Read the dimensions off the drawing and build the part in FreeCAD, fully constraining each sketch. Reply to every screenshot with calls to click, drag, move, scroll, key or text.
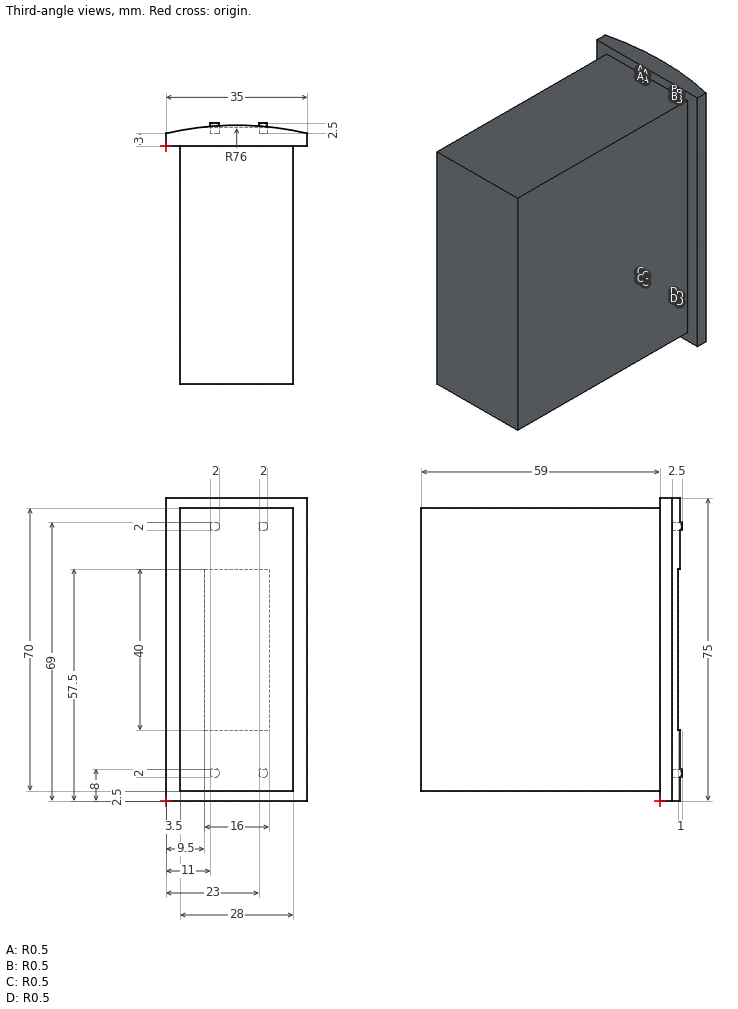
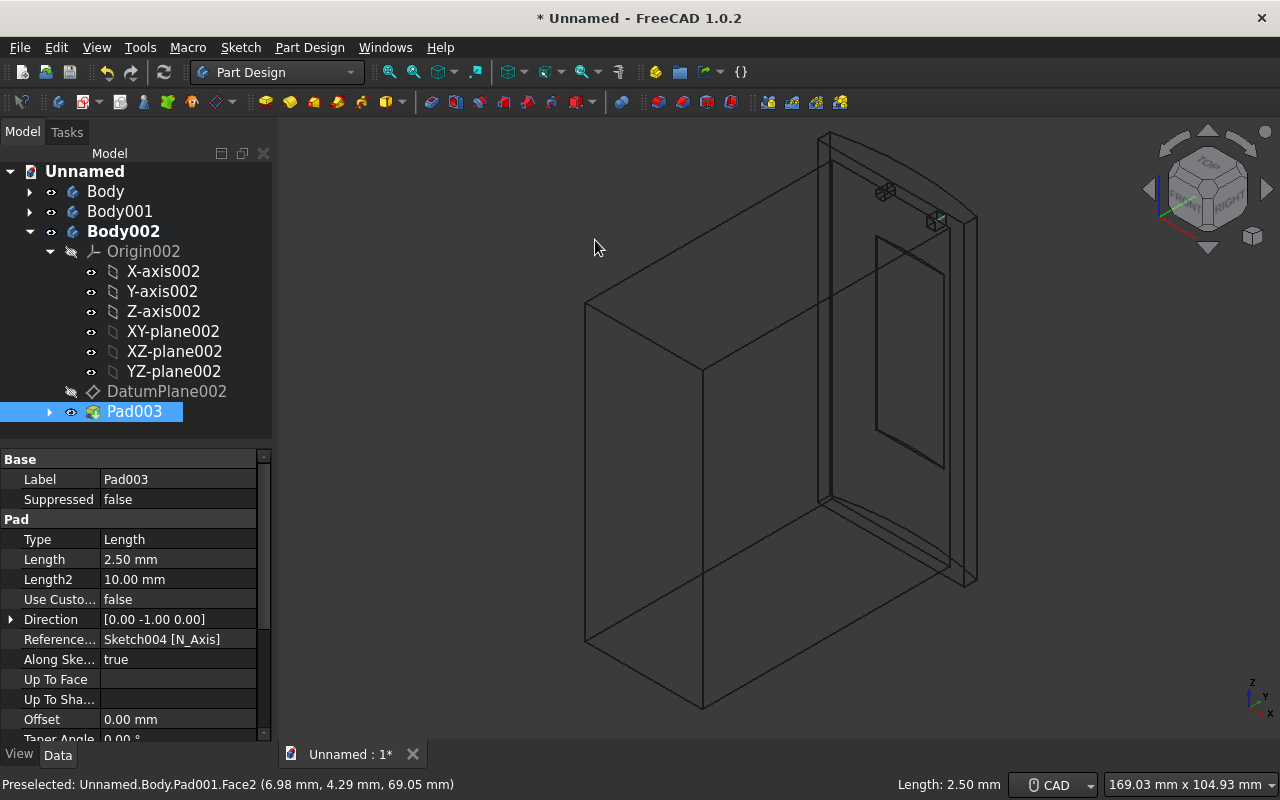
key(v)
key(f)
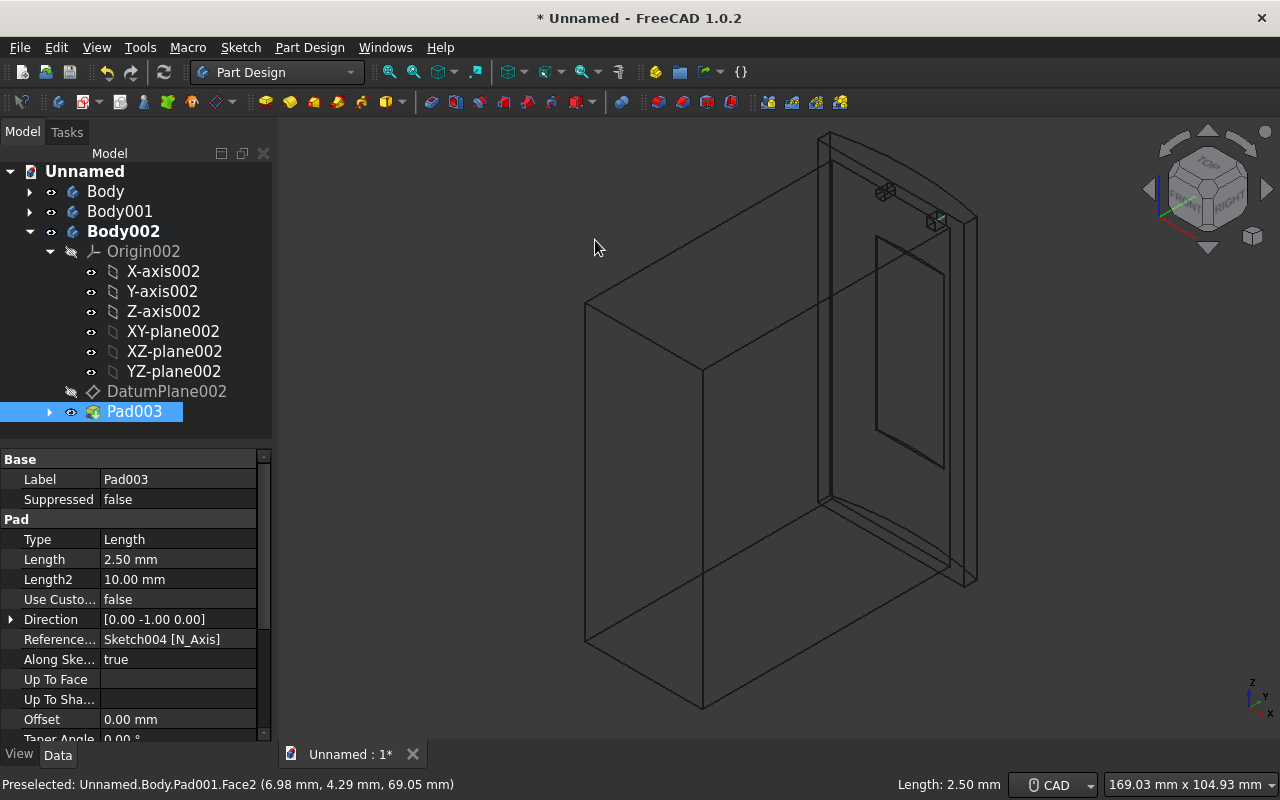
scroll(932, 213, up, 5)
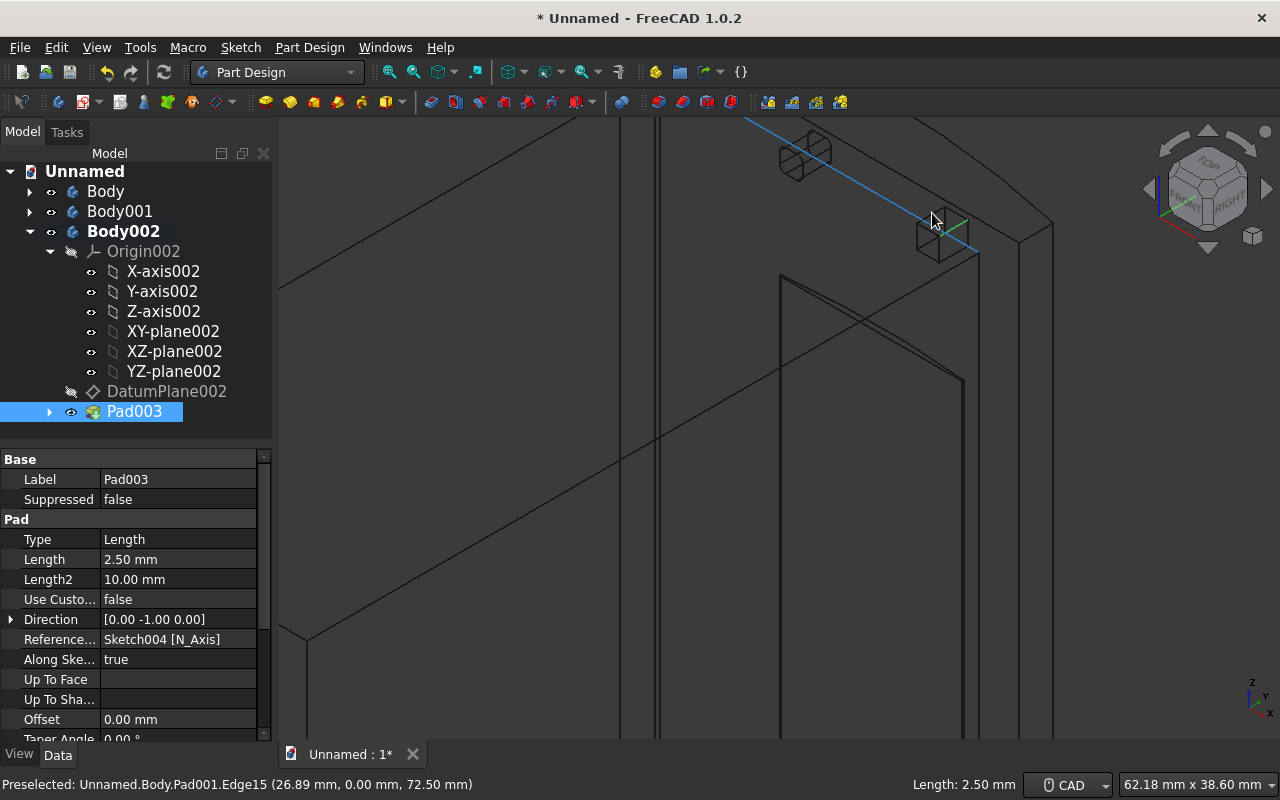
click(931, 214, ctrl)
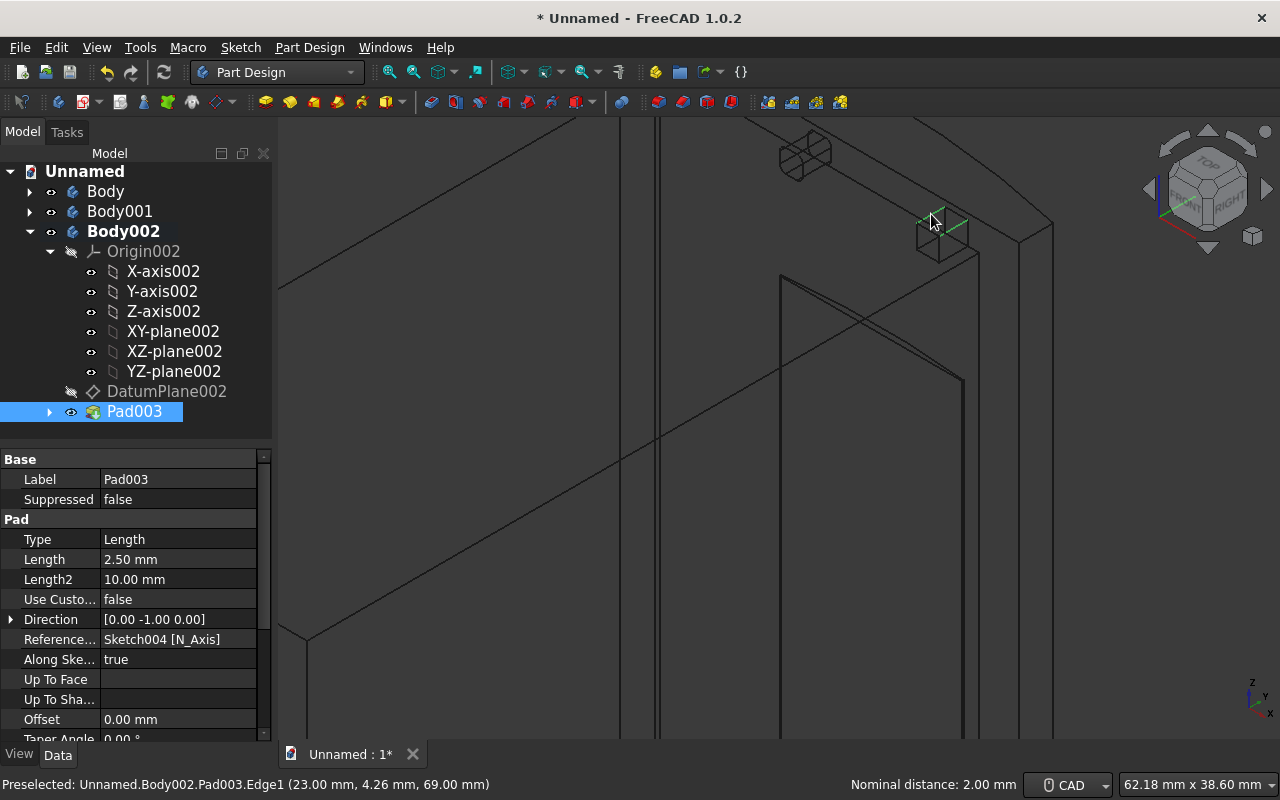
click(954, 253, ctrl)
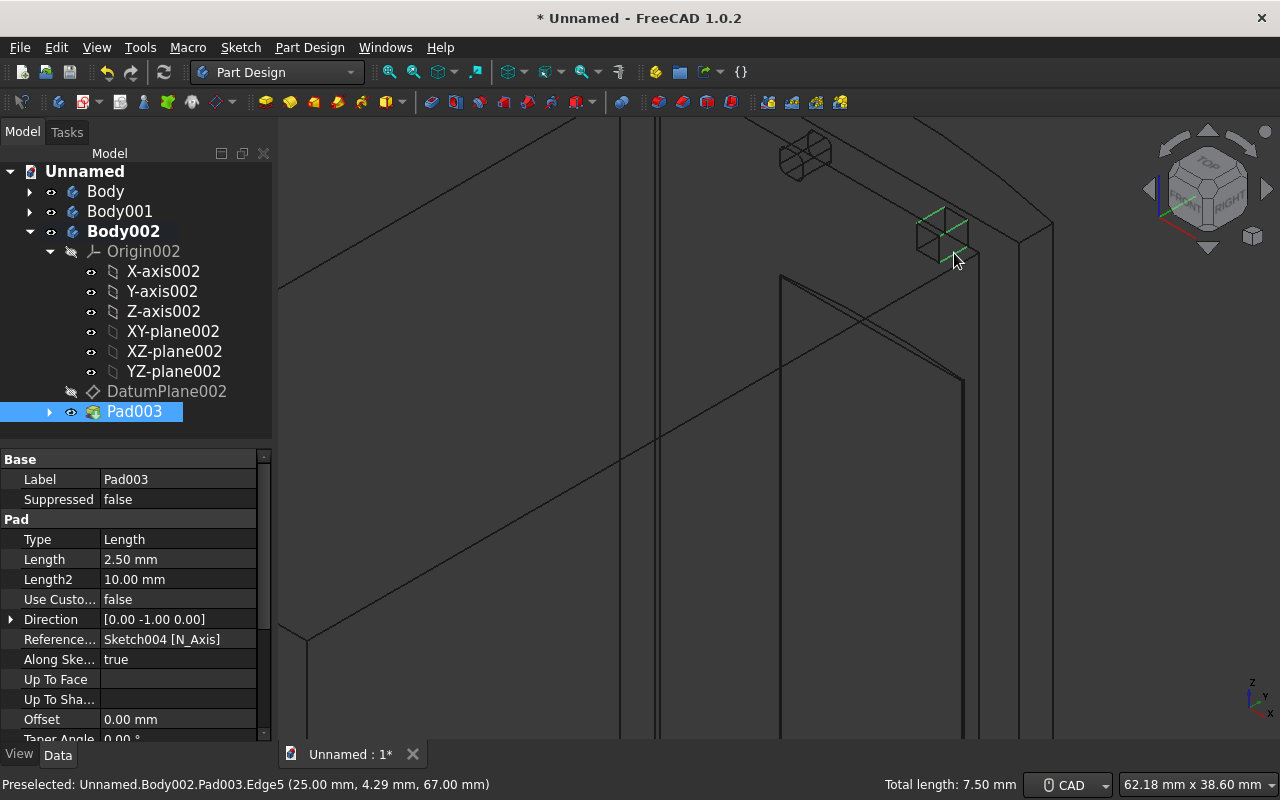
click(931, 240, ctrl)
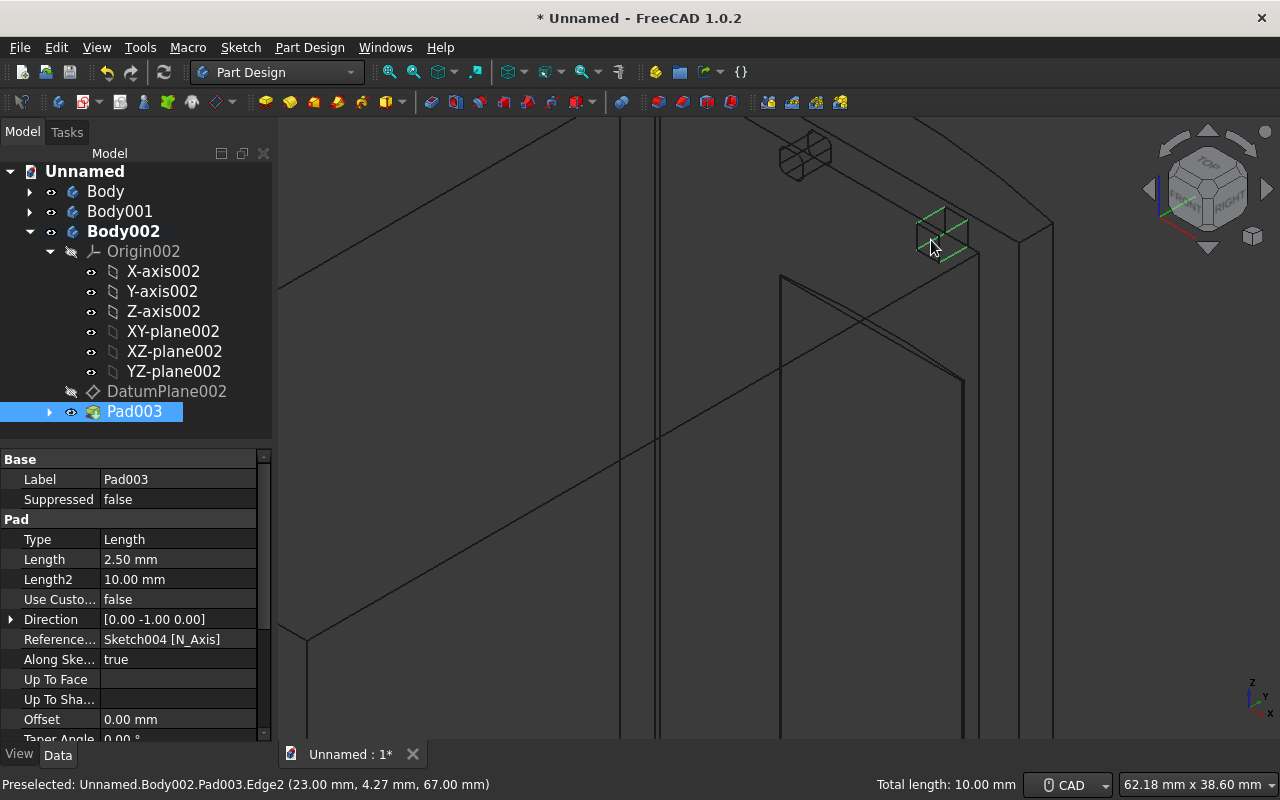
key(v)
key(1)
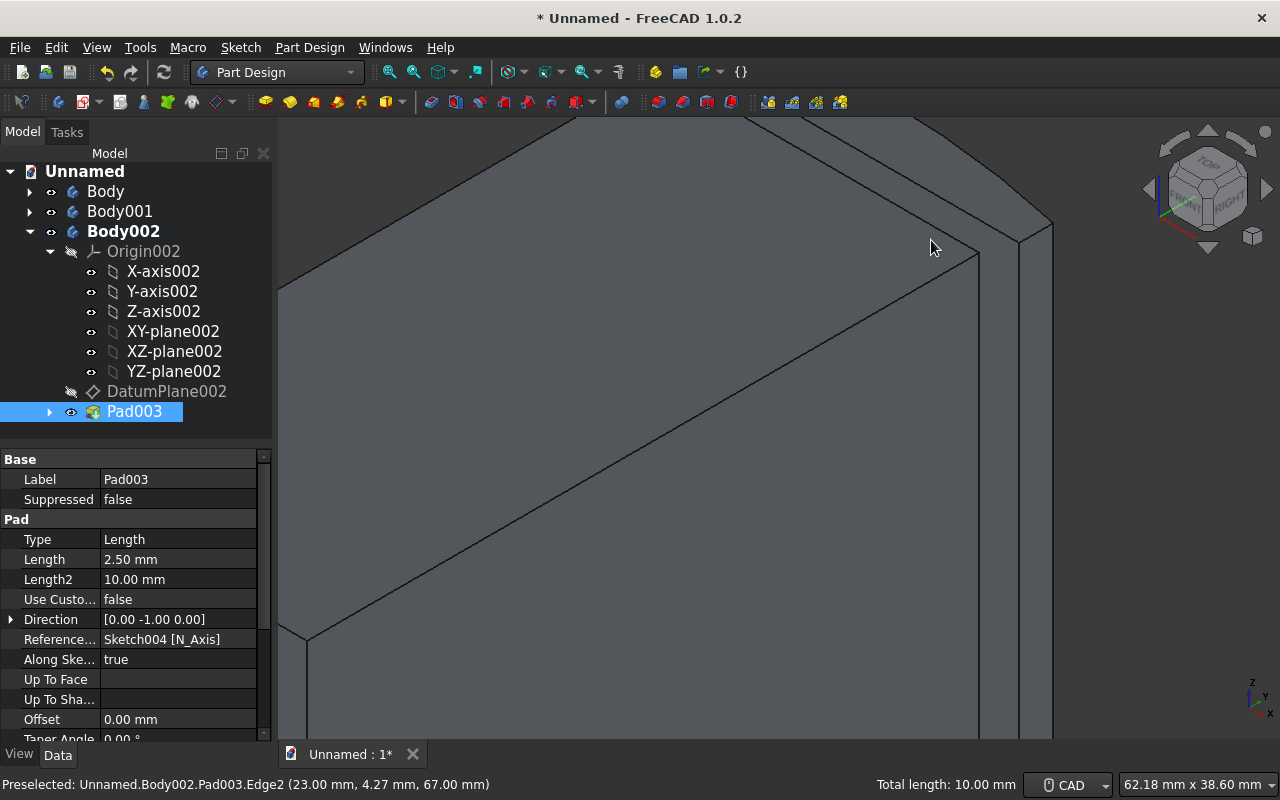
click(660, 102)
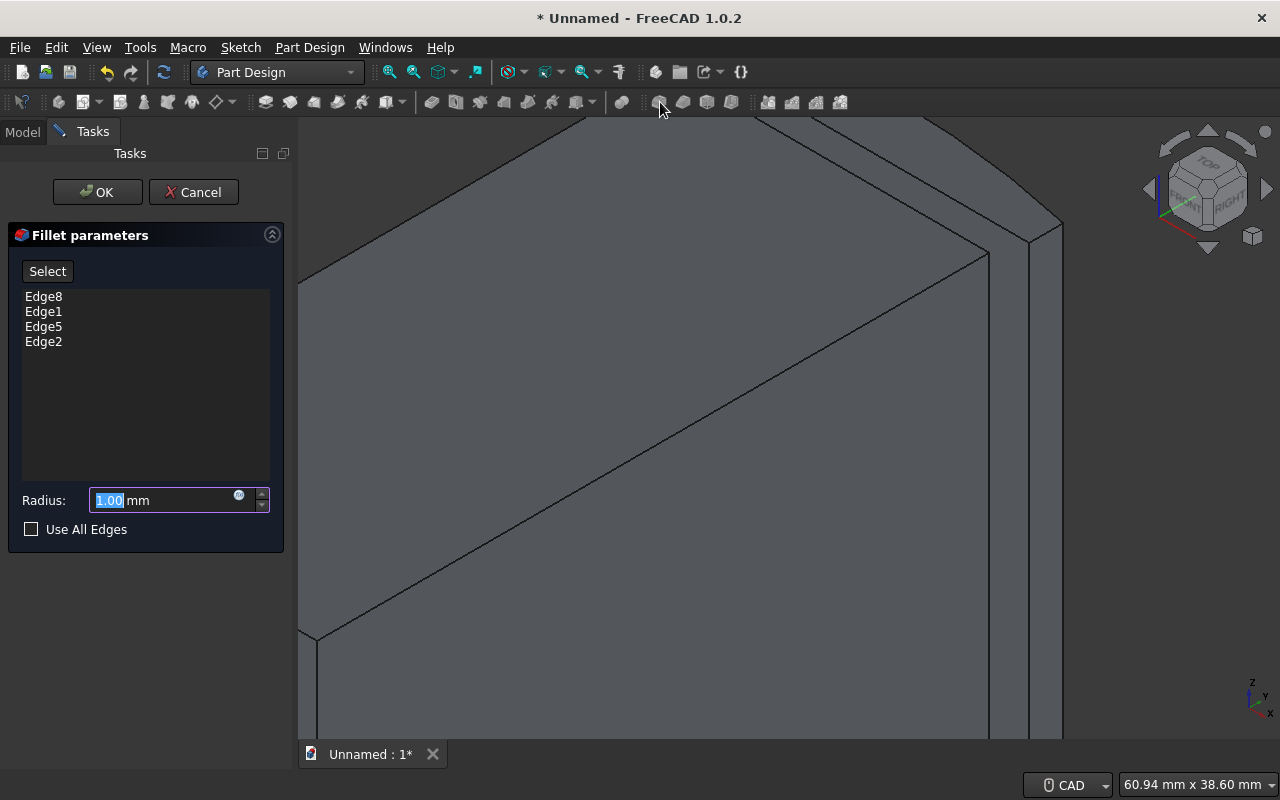
text(0.5)
key(Tab)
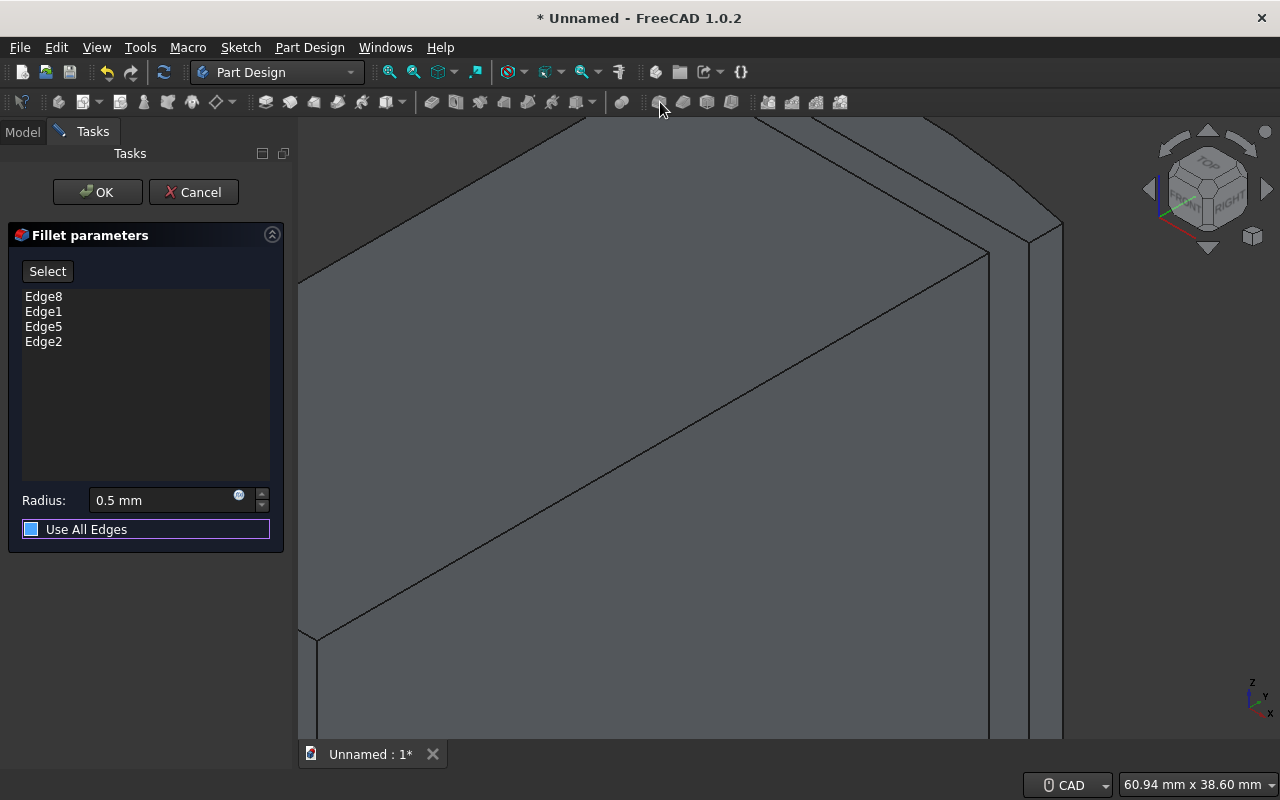
click(98, 192)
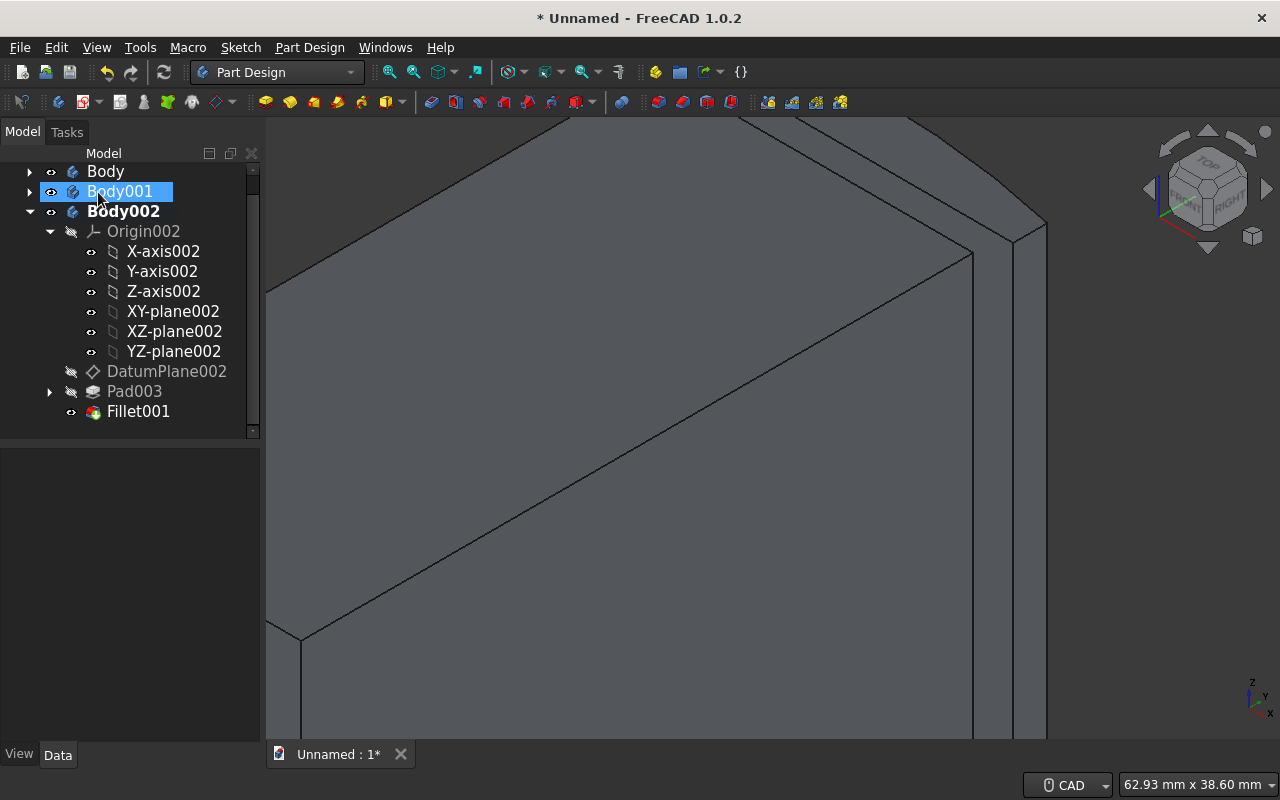
key(v)
key(f)